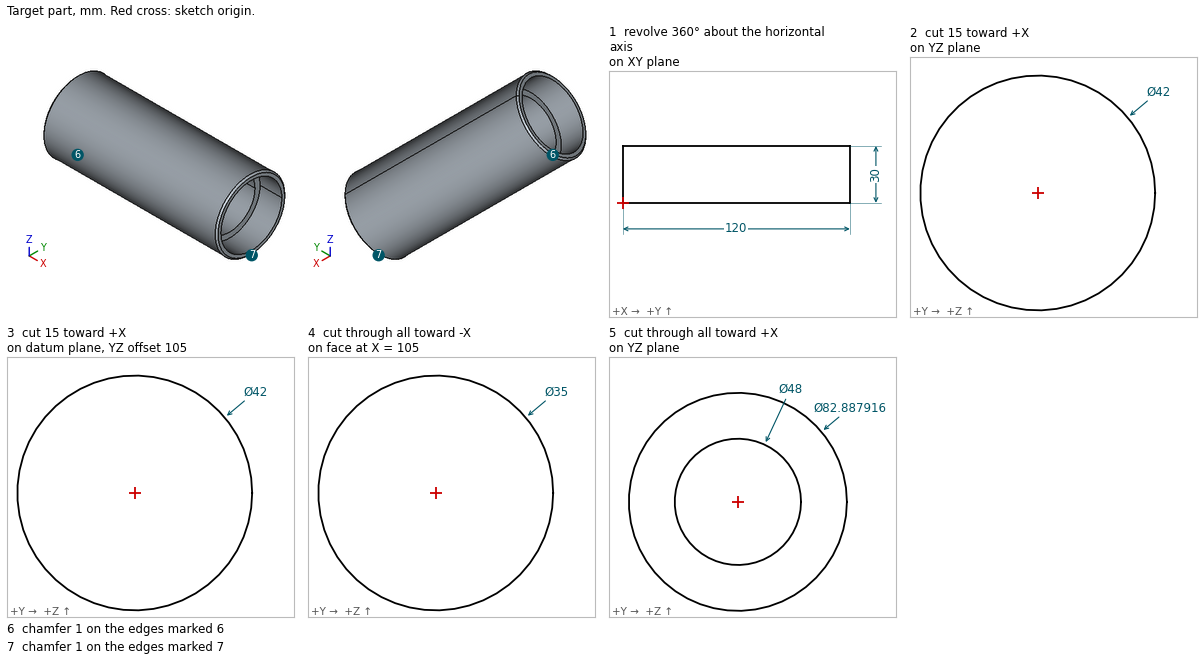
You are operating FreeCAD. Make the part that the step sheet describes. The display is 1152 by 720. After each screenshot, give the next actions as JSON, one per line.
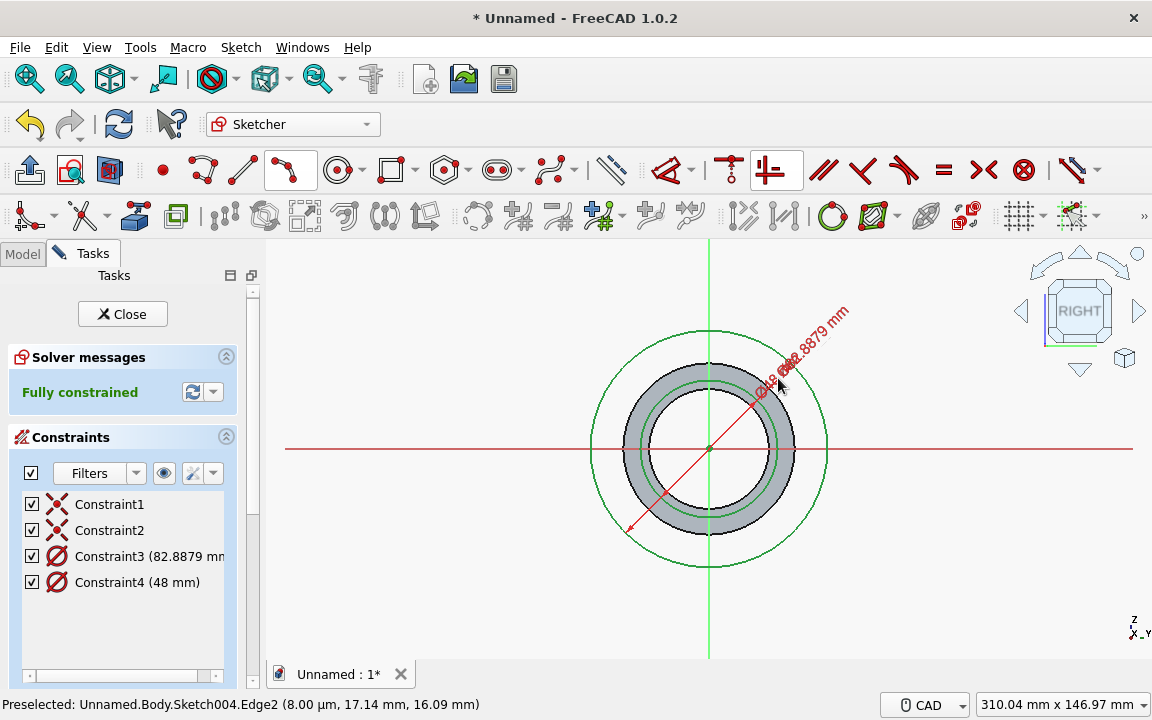
{"action": "left_click", "coordinate": [123, 314]}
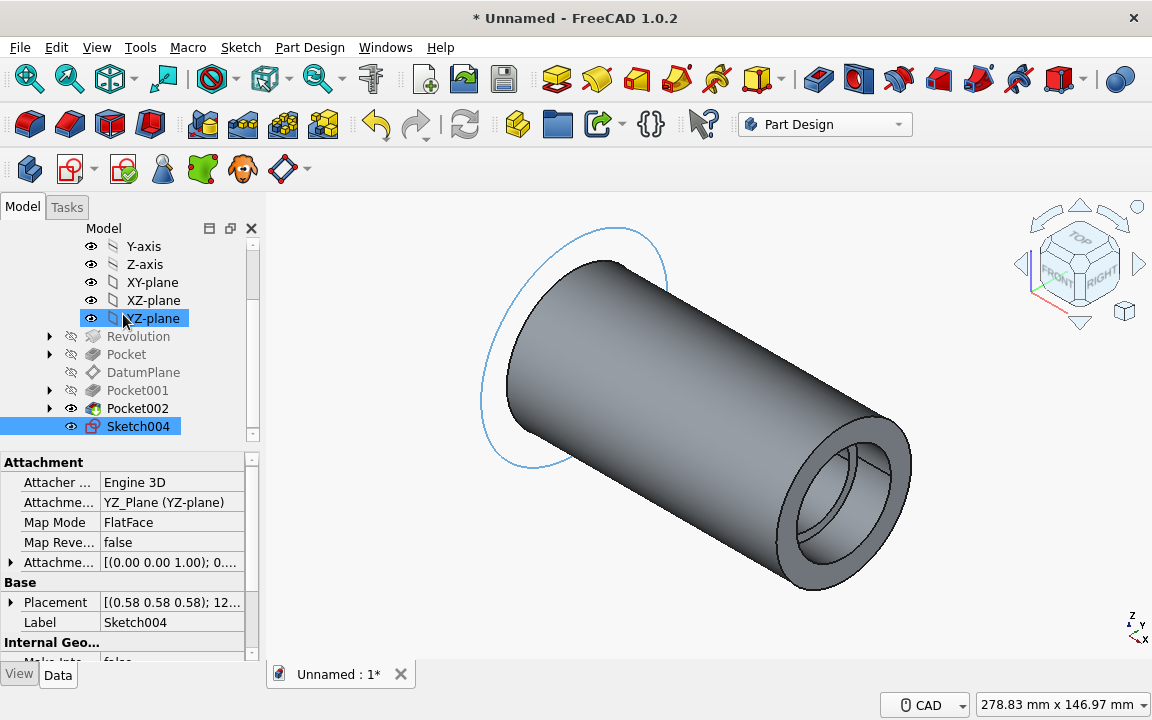
{"action": "left_click", "coordinate": [820, 80]}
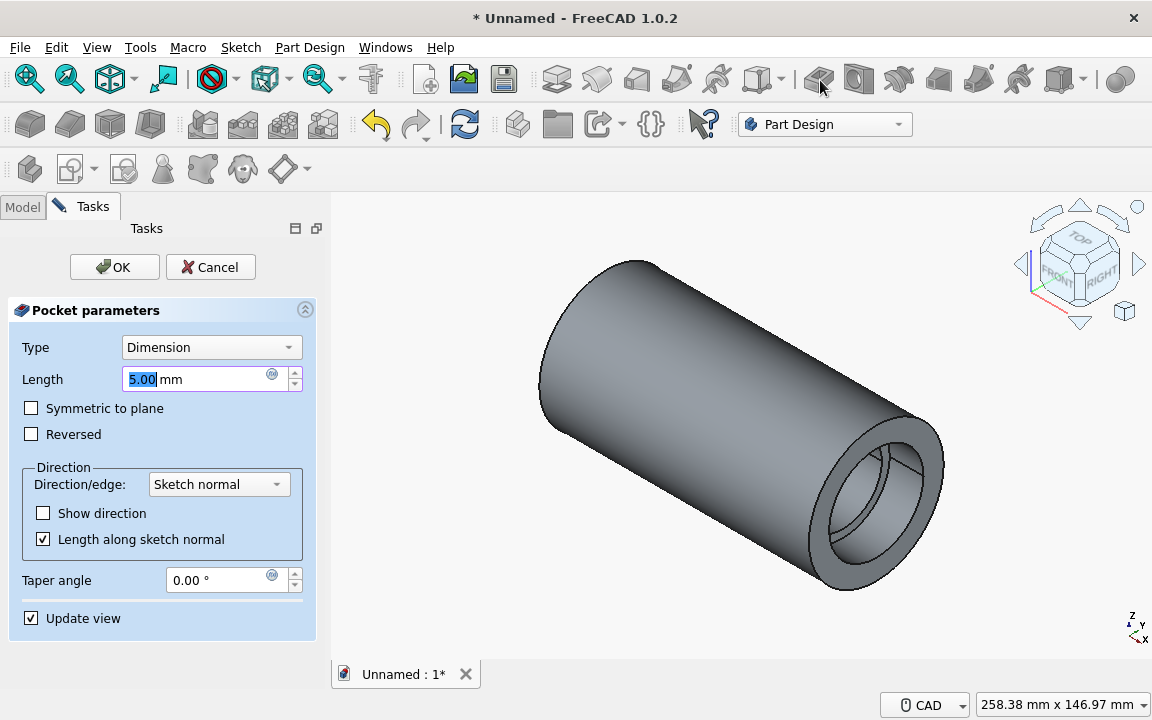
{"action": "left_click", "coordinate": [212, 348]}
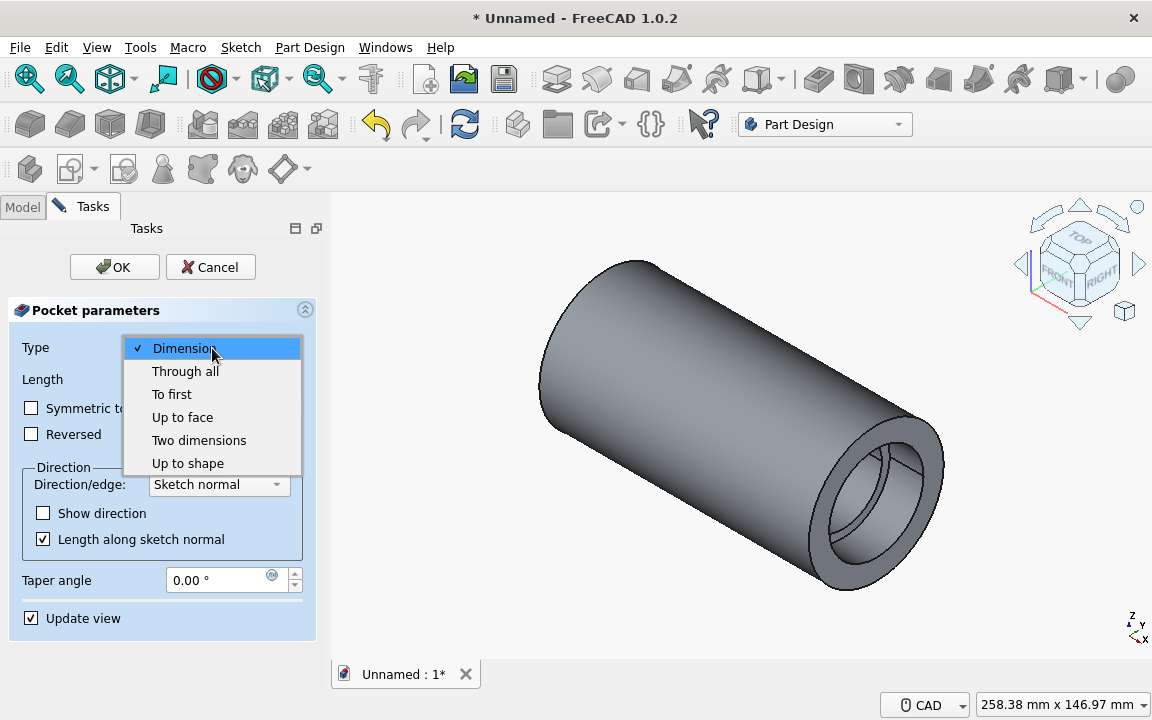
{"action": "left_click", "coordinate": [212, 372]}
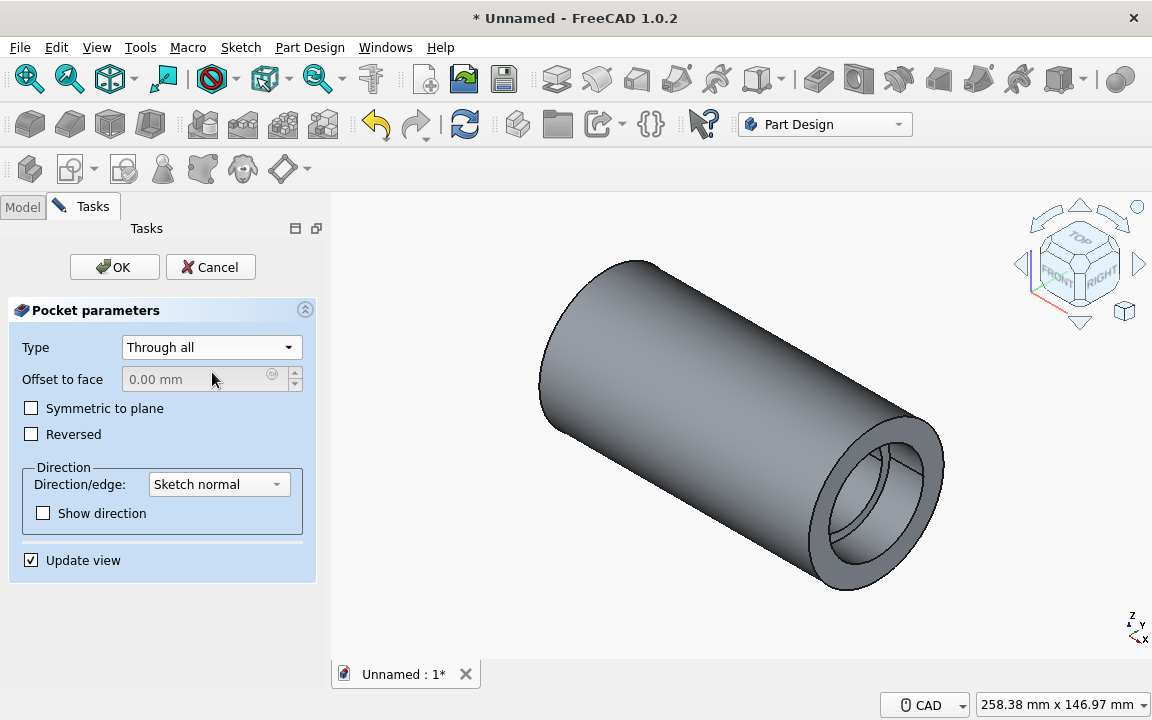
{"action": "left_click", "coordinate": [30, 434]}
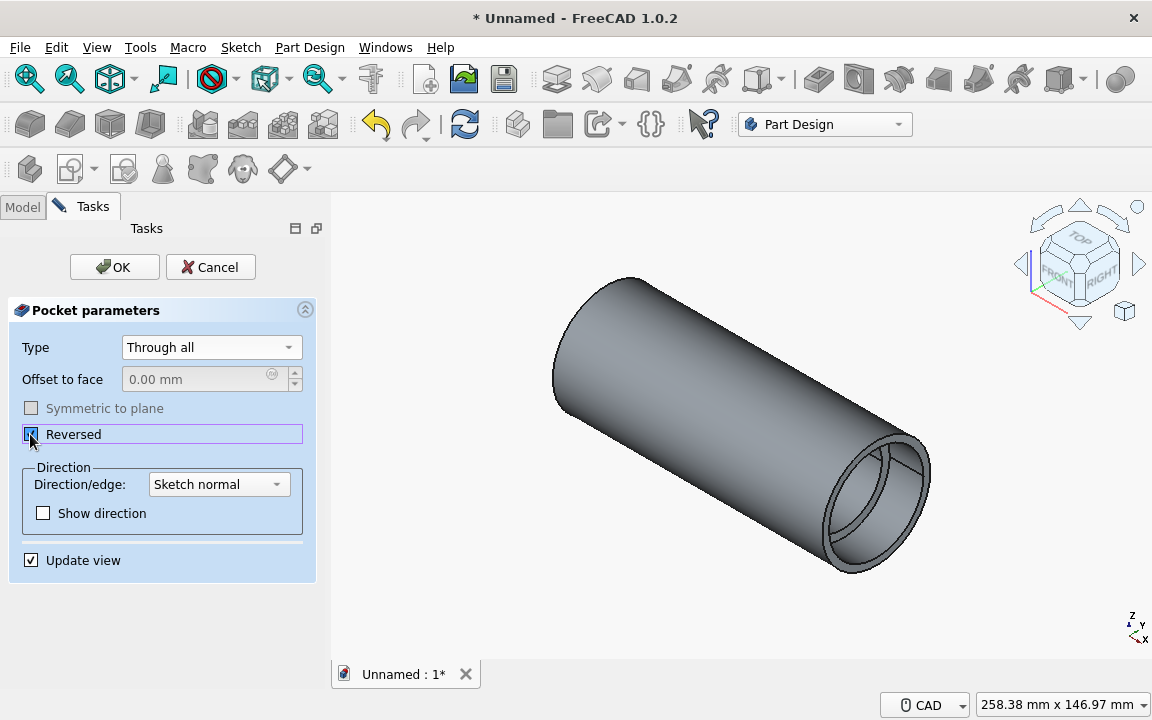
{"action": "left_click", "coordinate": [115, 267]}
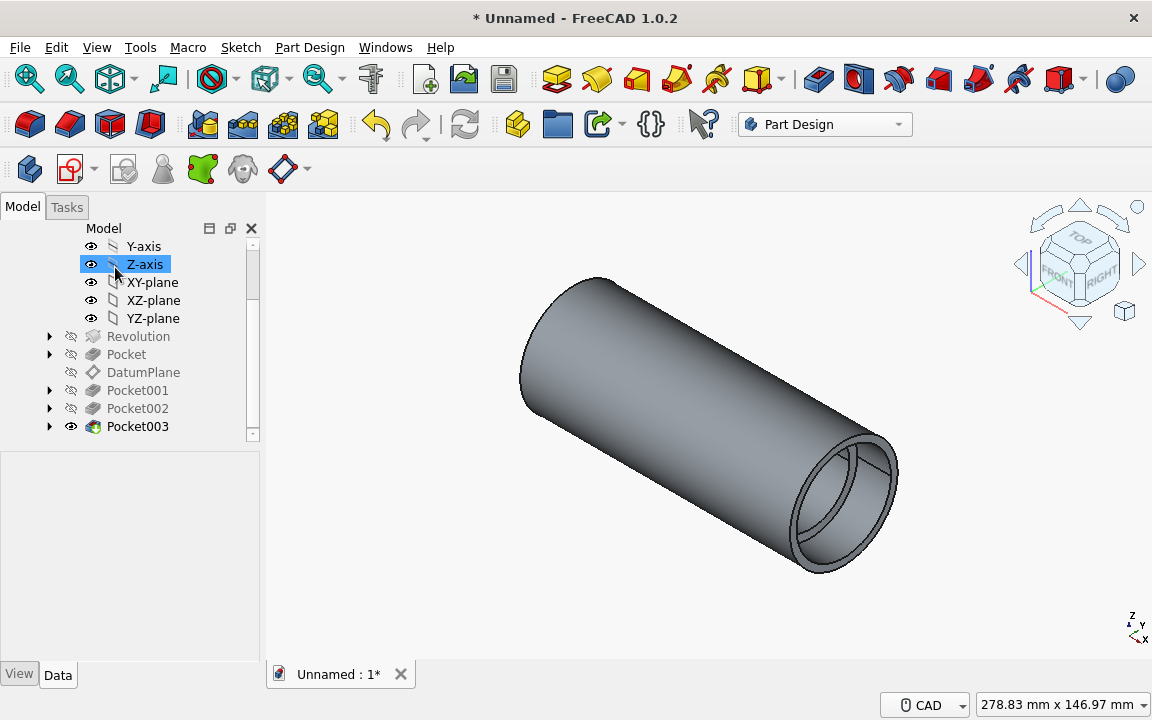
{"action": "key", "text": "2"}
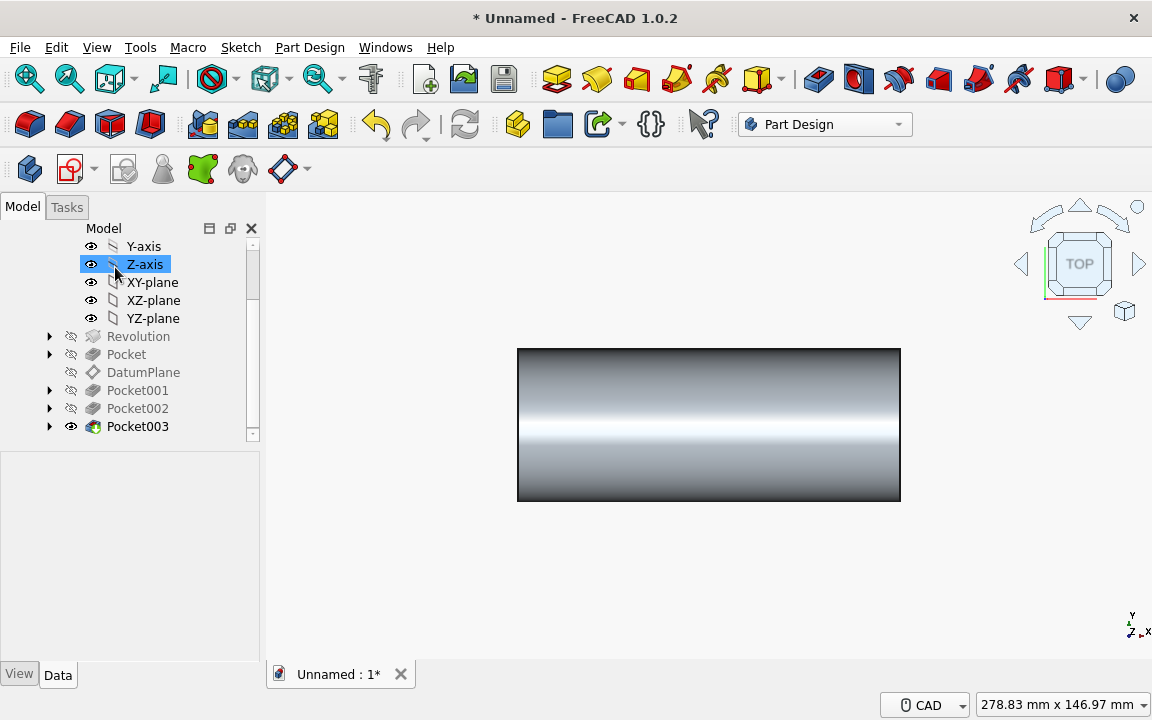
{"action": "left_click", "coordinate": [30, 80]}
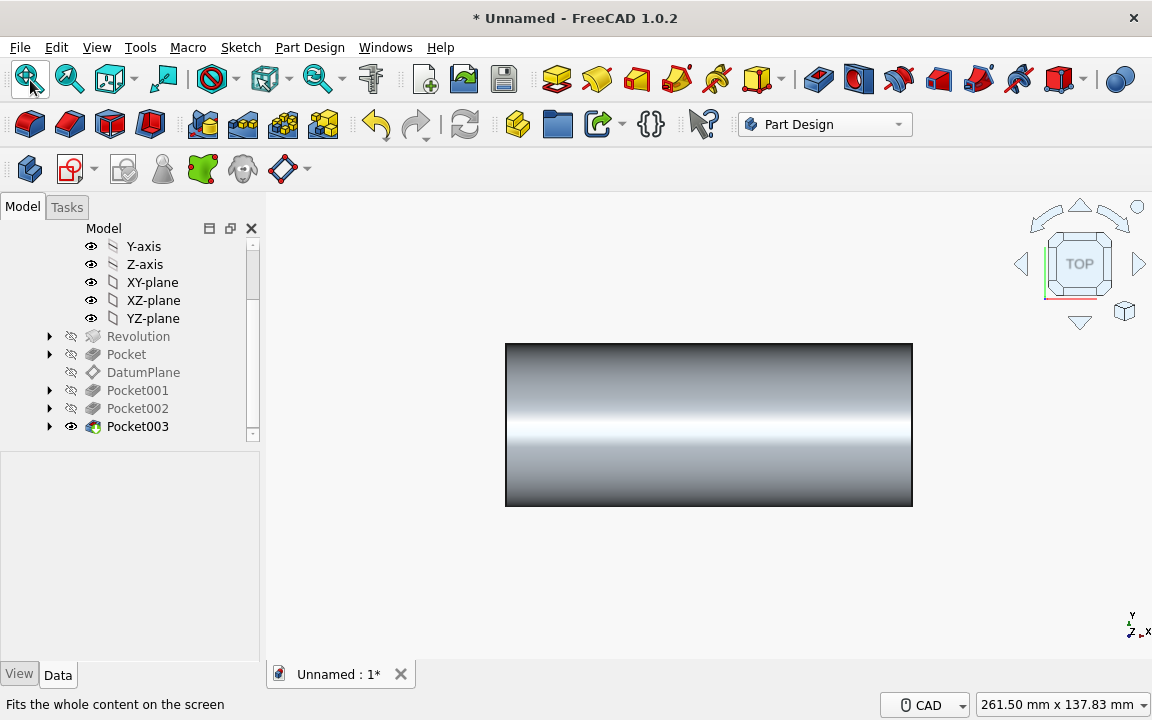
{"action": "left_click", "coordinate": [506, 490]}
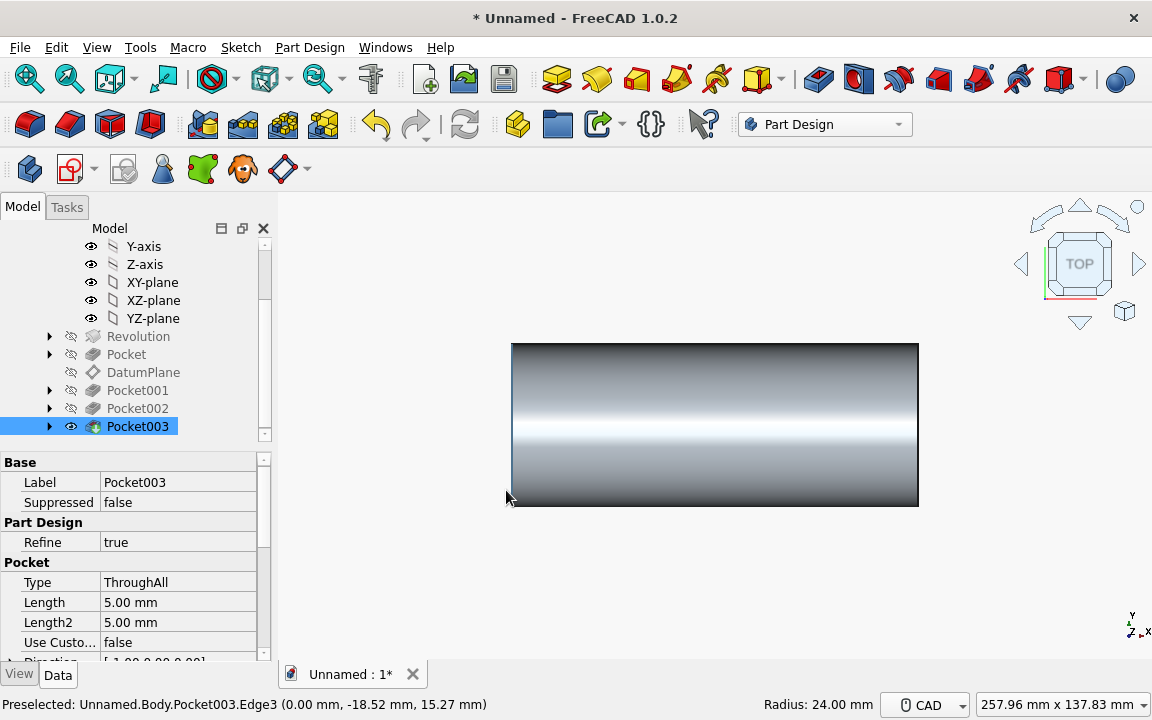
{"action": "left_click", "coordinate": [70, 124]}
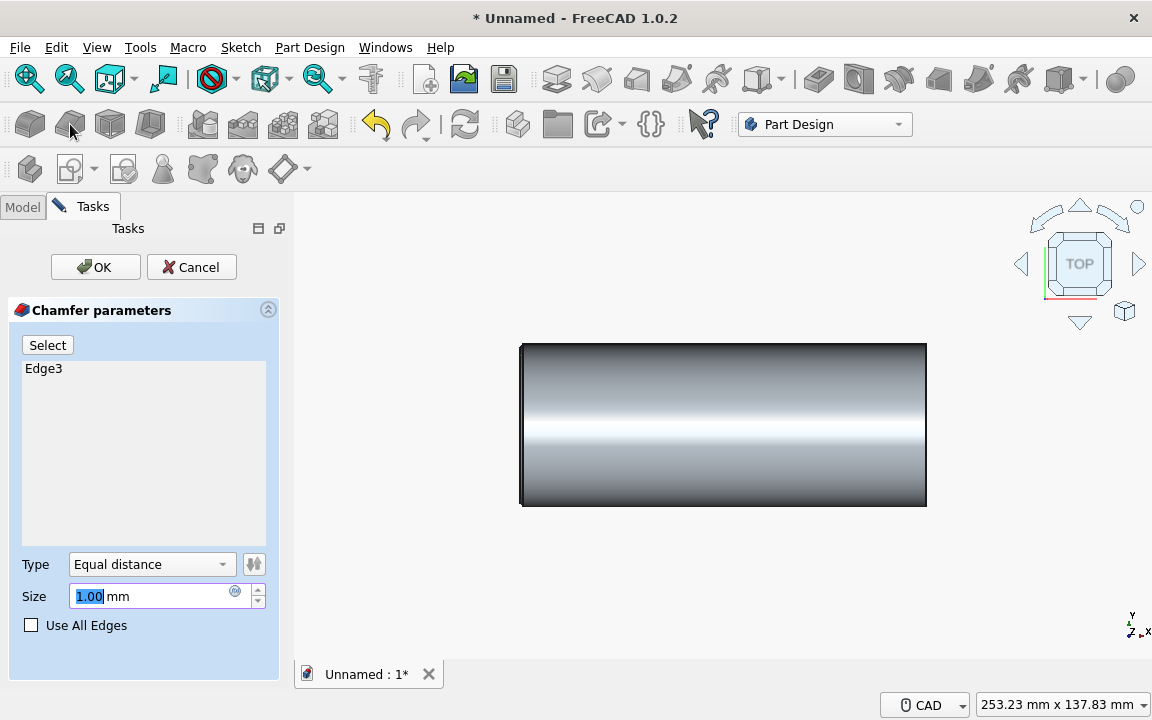
{"action": "type", "text": "1"}
{"action": "key", "text": "Tab"}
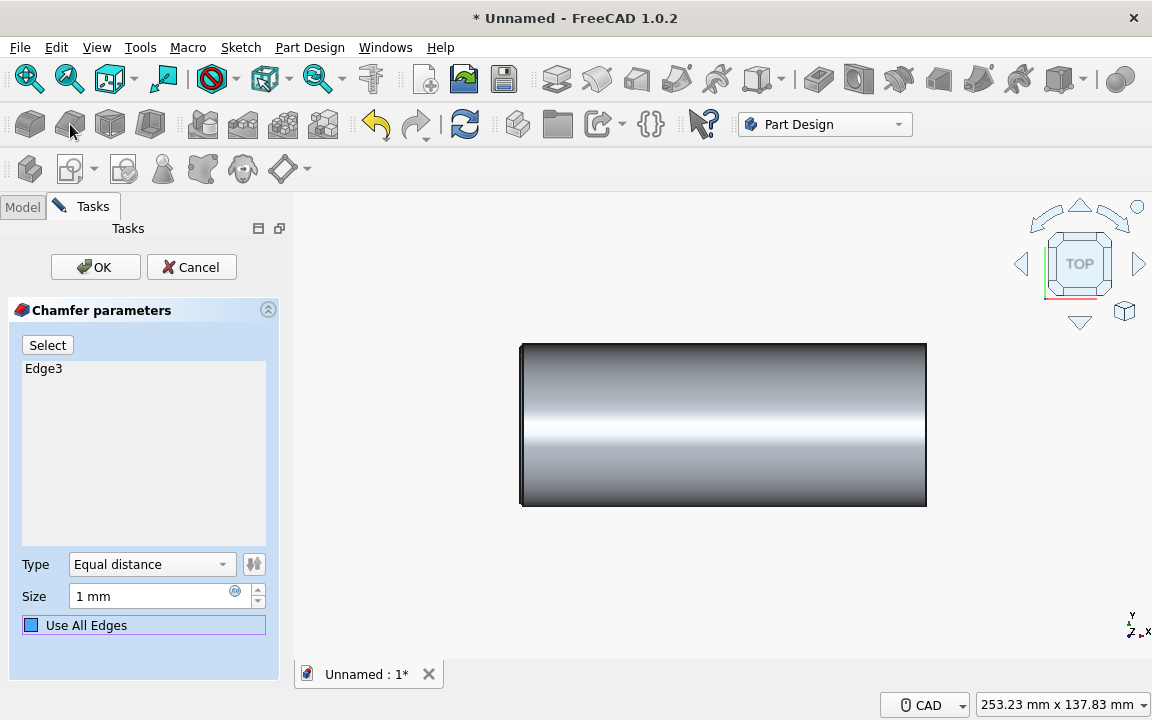
{"action": "left_click", "coordinate": [96, 267]}